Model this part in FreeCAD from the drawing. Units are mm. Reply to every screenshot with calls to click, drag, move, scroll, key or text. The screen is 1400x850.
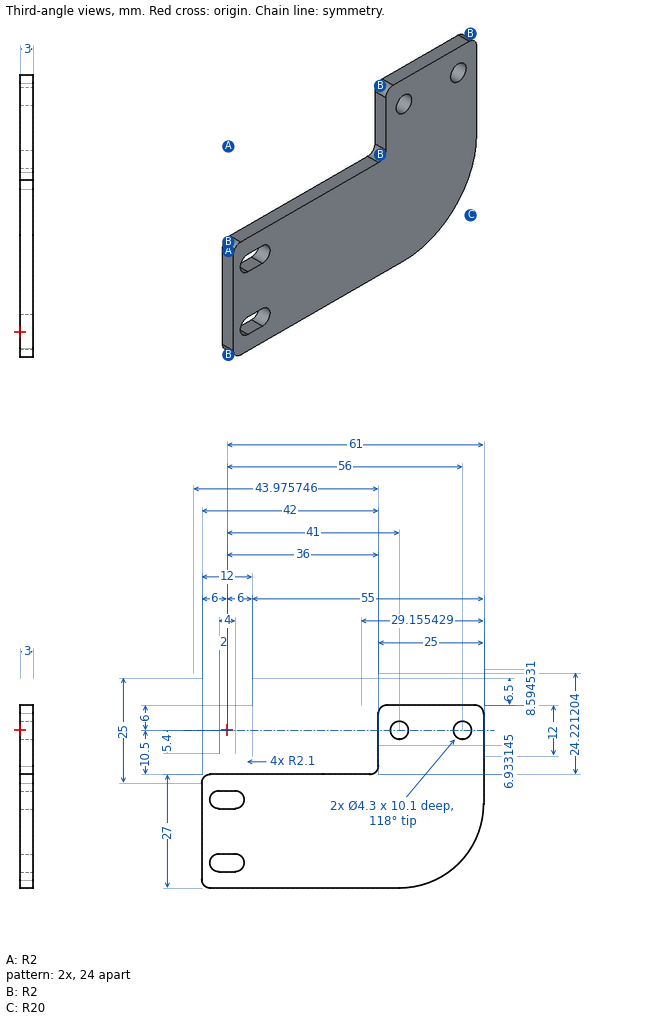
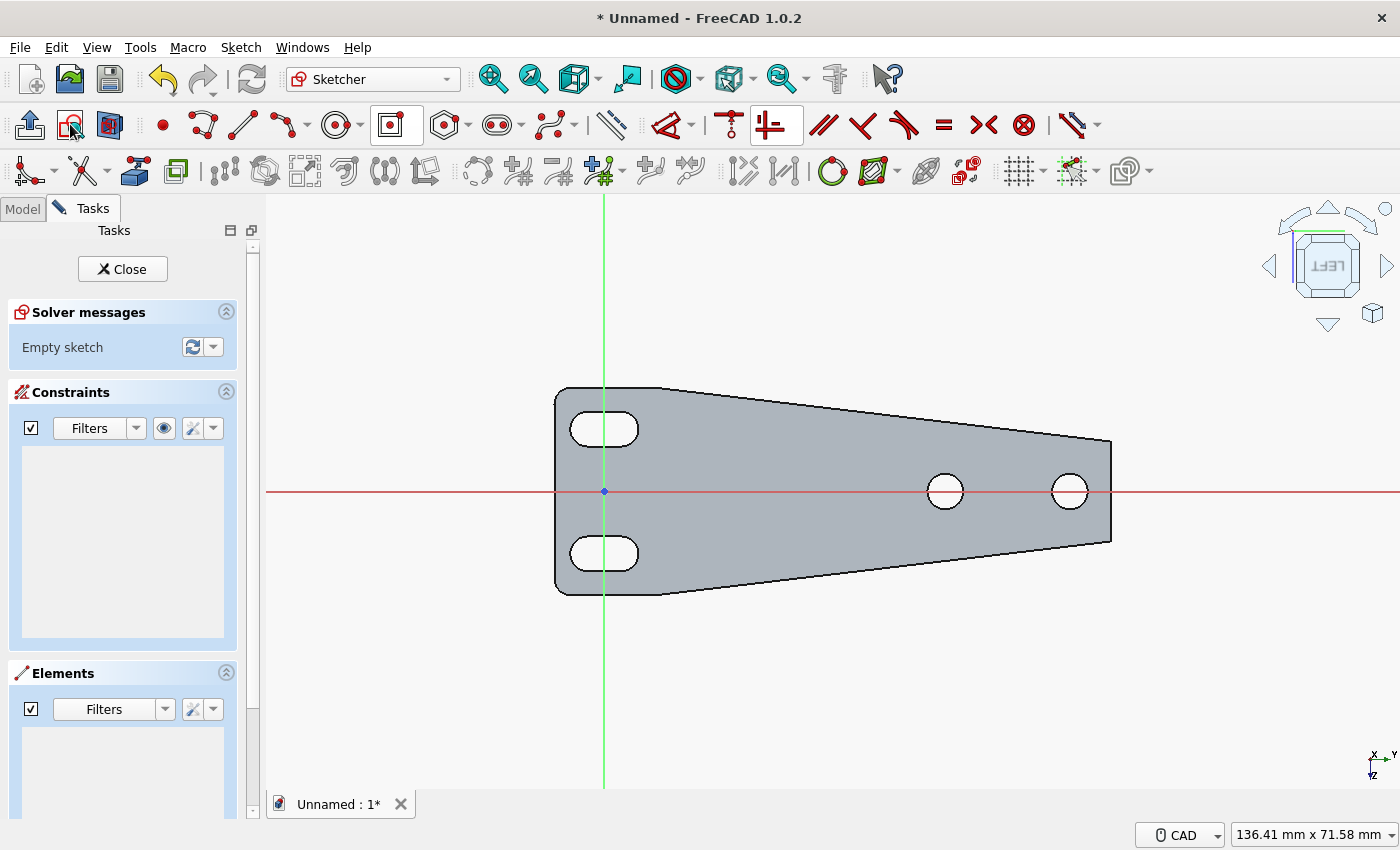
scroll(455, 761, down, 1)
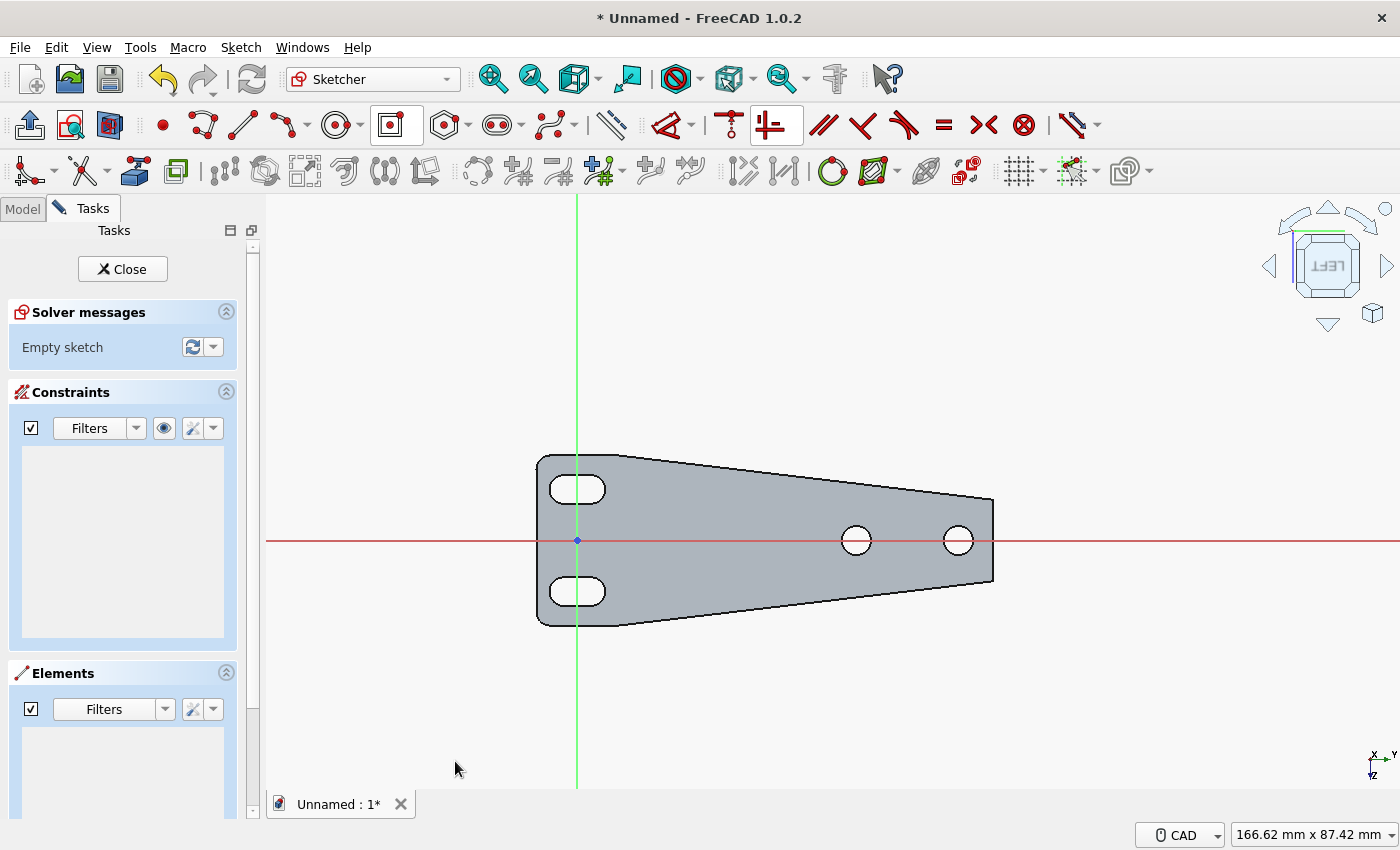
scroll(765, 253, up, 2)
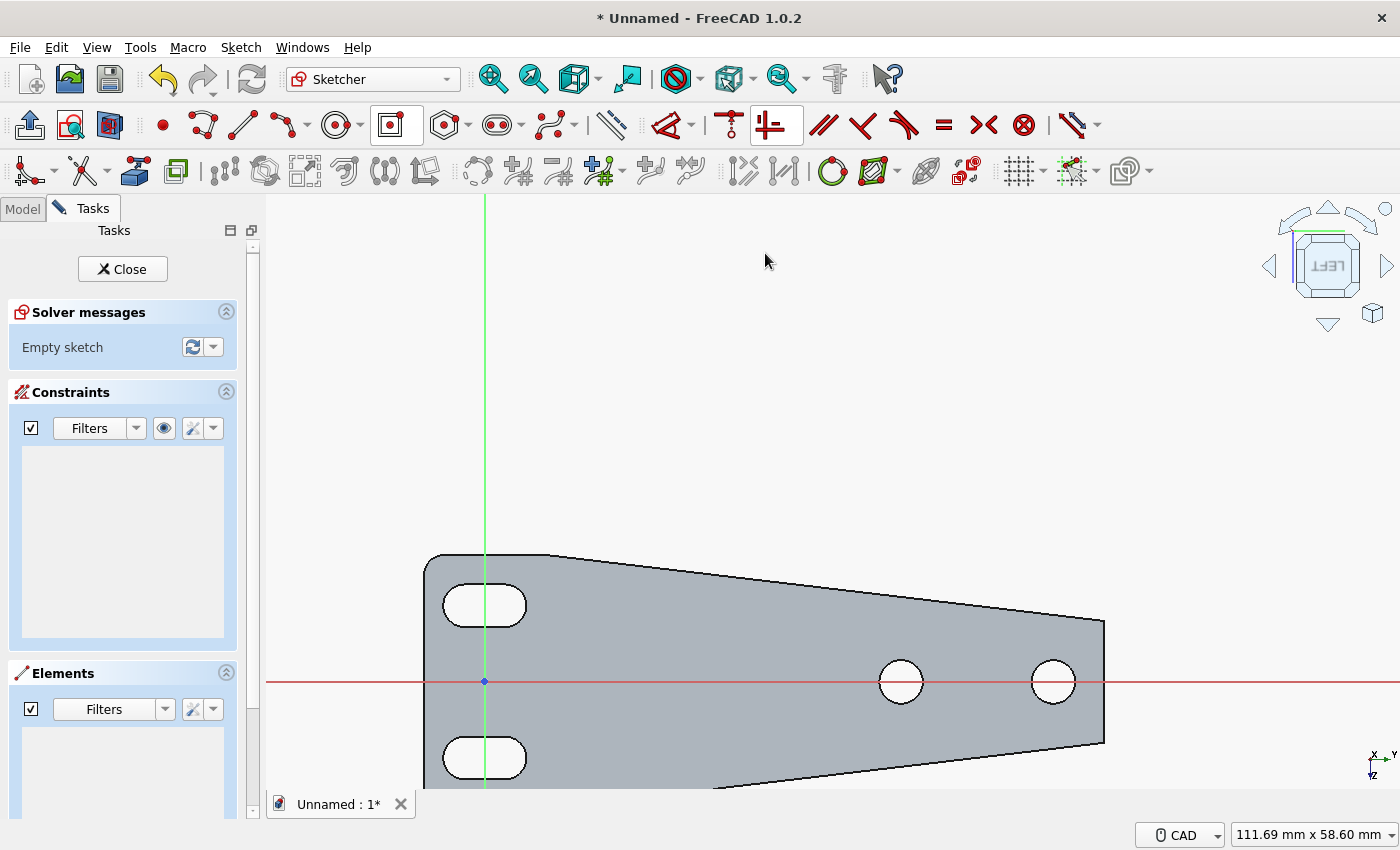
click(204, 126)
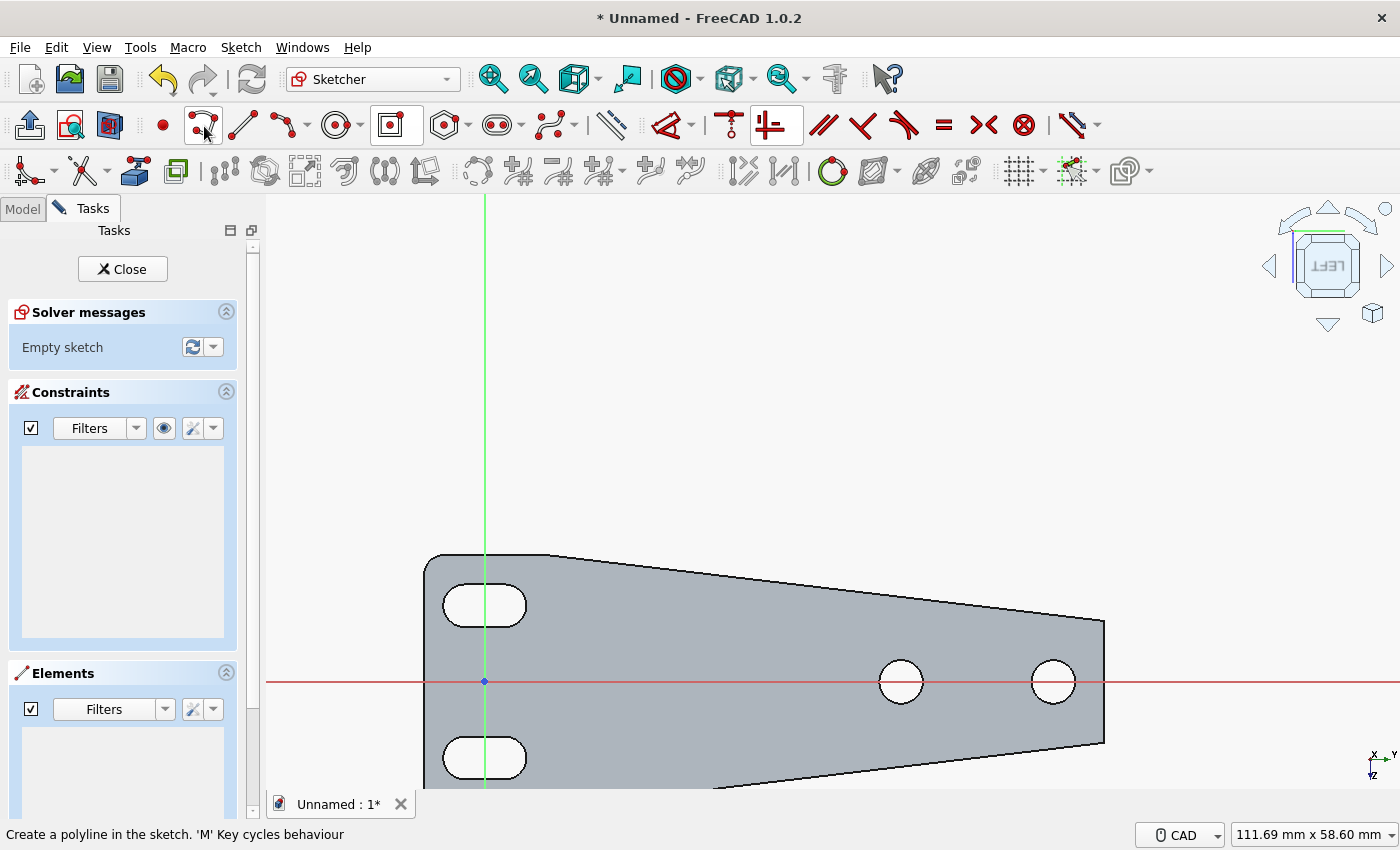
click(424, 575)
click(850, 575)
click(850, 646)
click(1104, 646)
click(1104, 301)
click(424, 301)
click(424, 576)
key(Escape)
key(Escape)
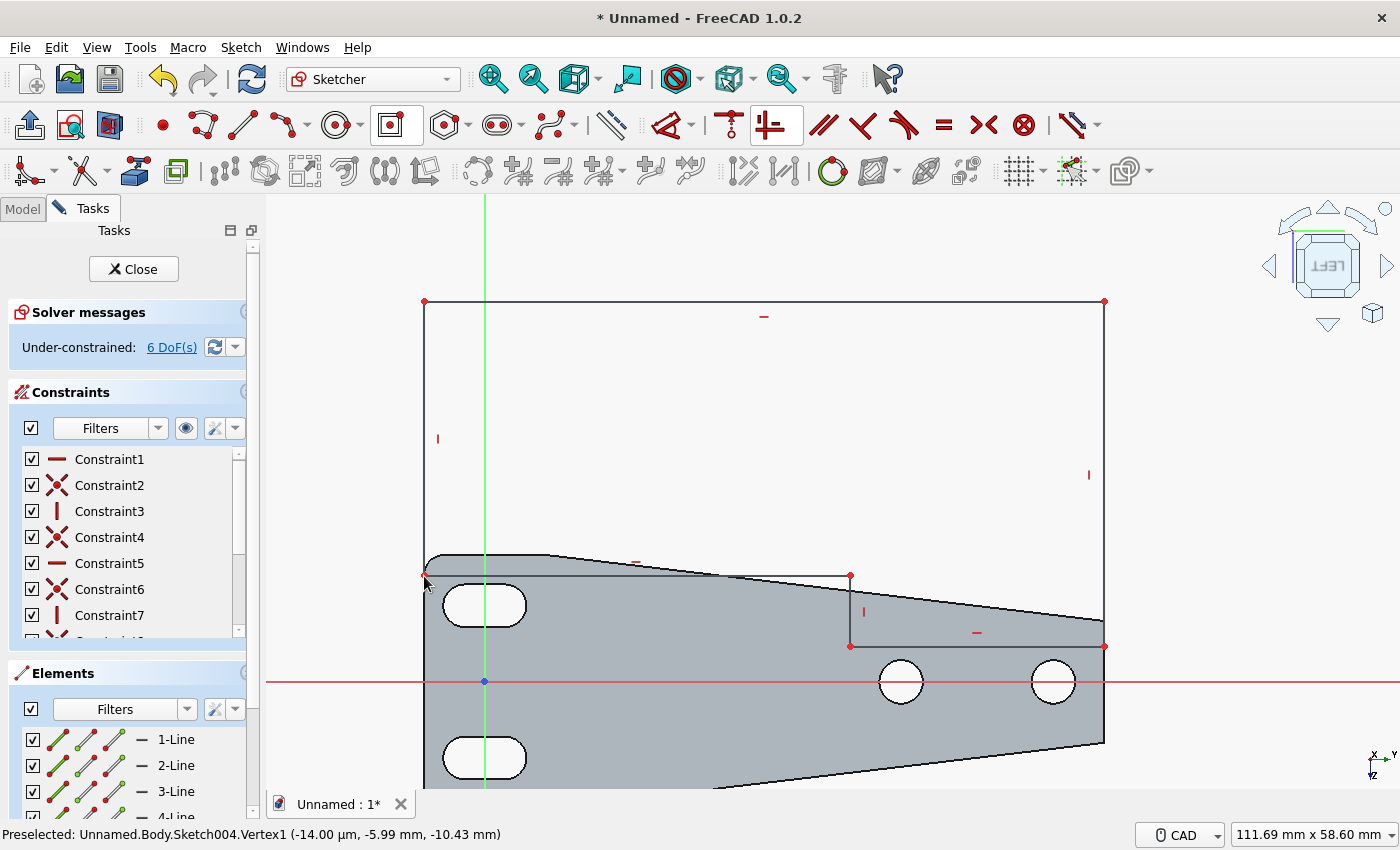
click(666, 126)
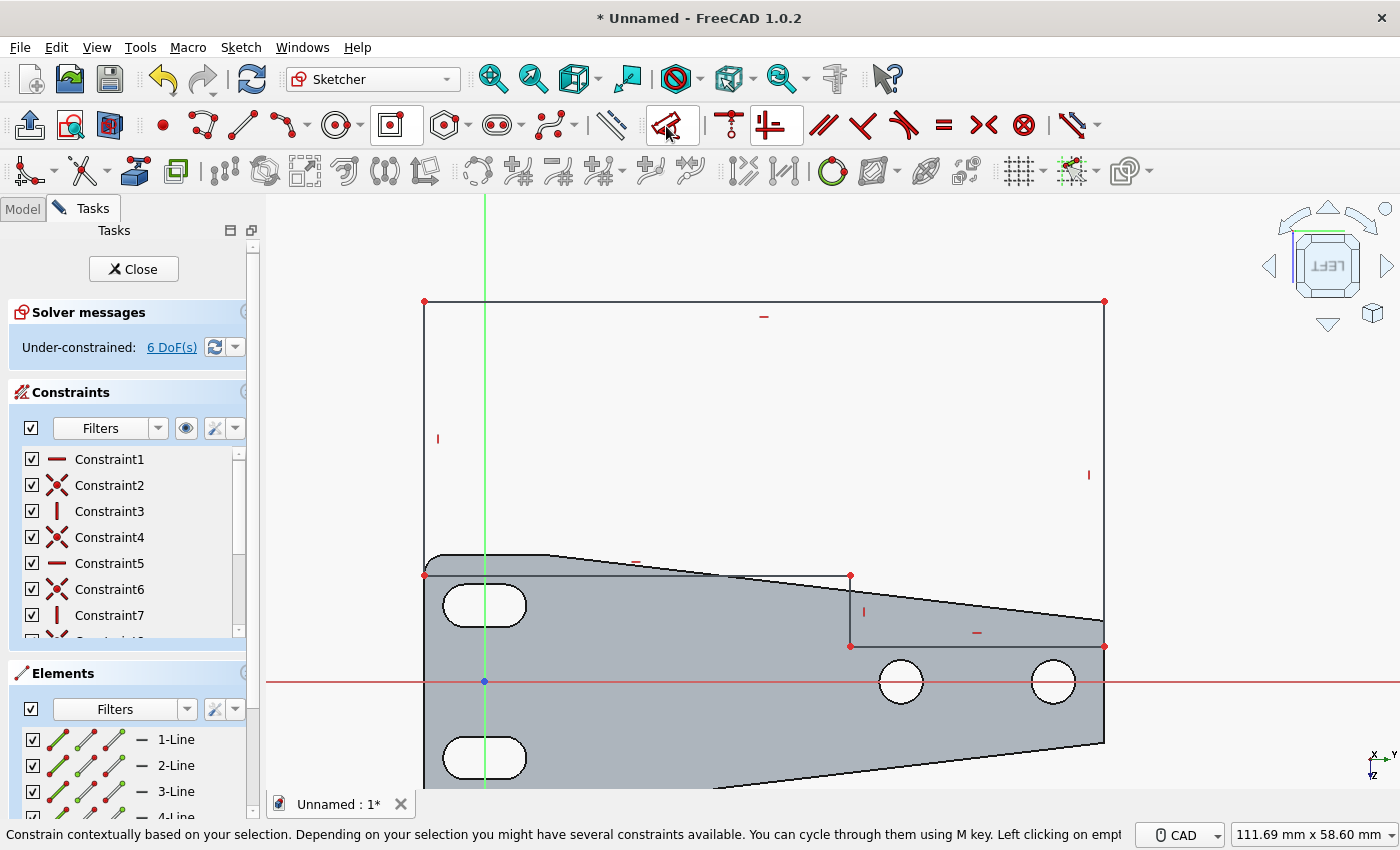
click(552, 576)
click(637, 610)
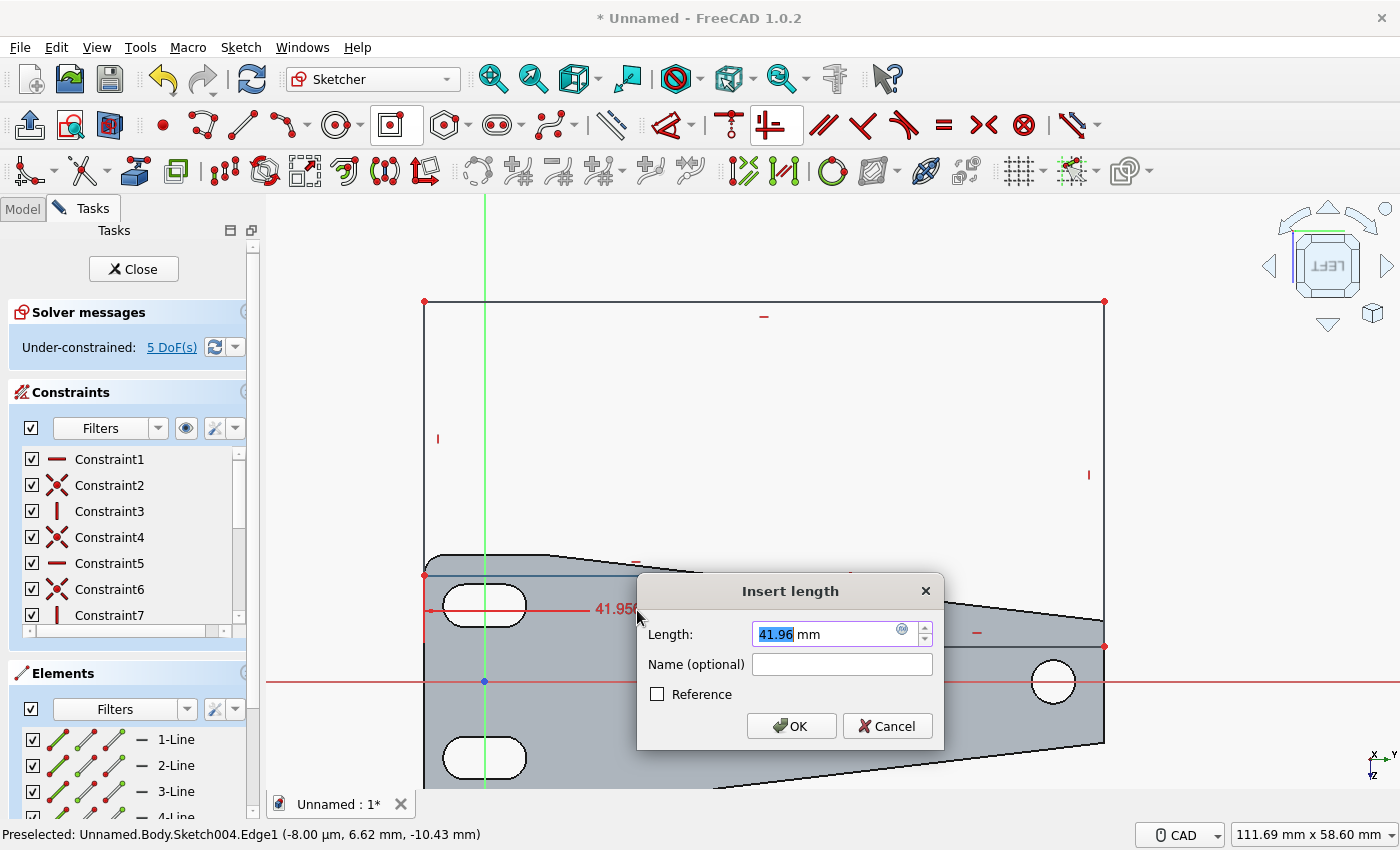
text(42)
key(Return)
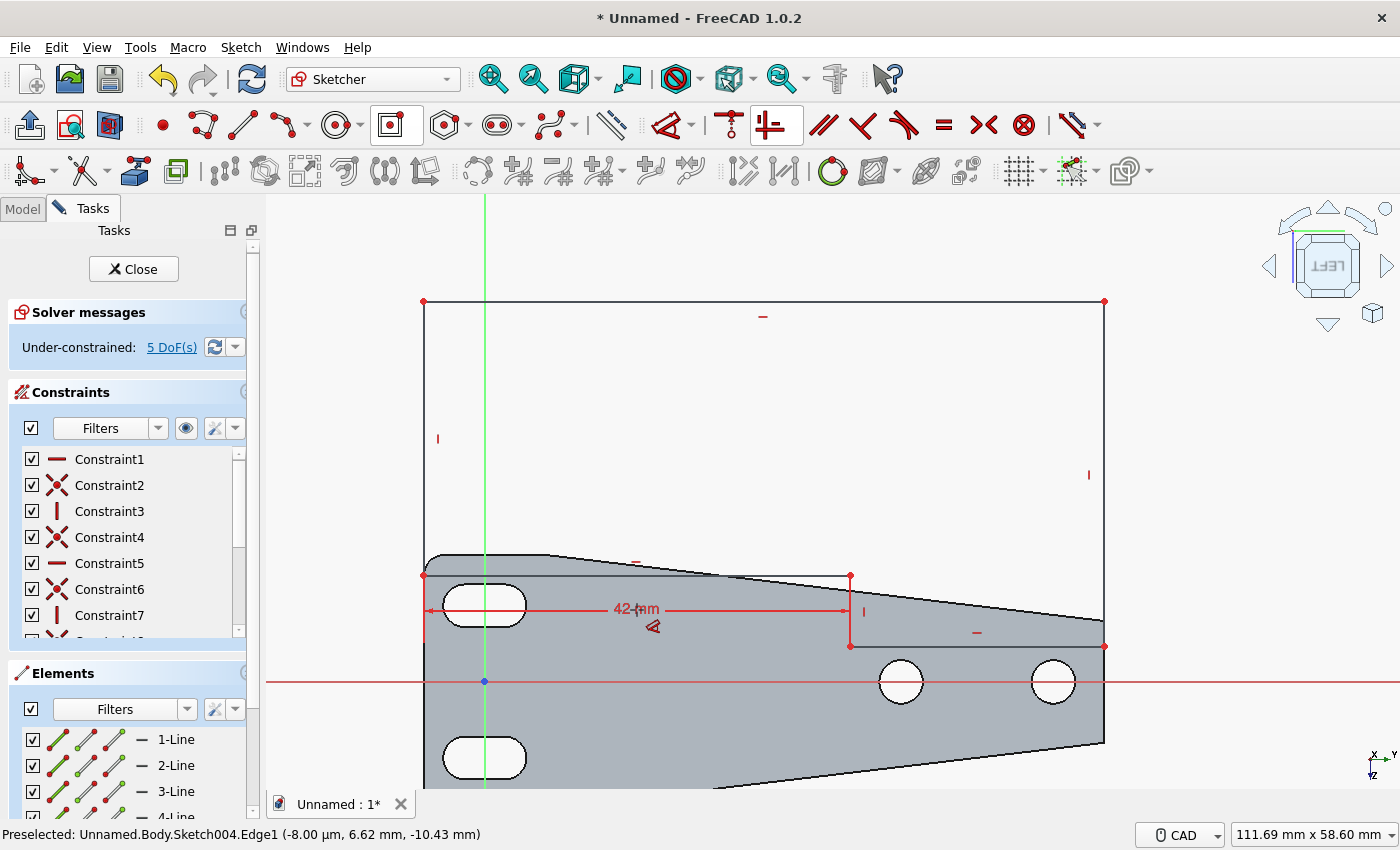
click(926, 647)
click(977, 613)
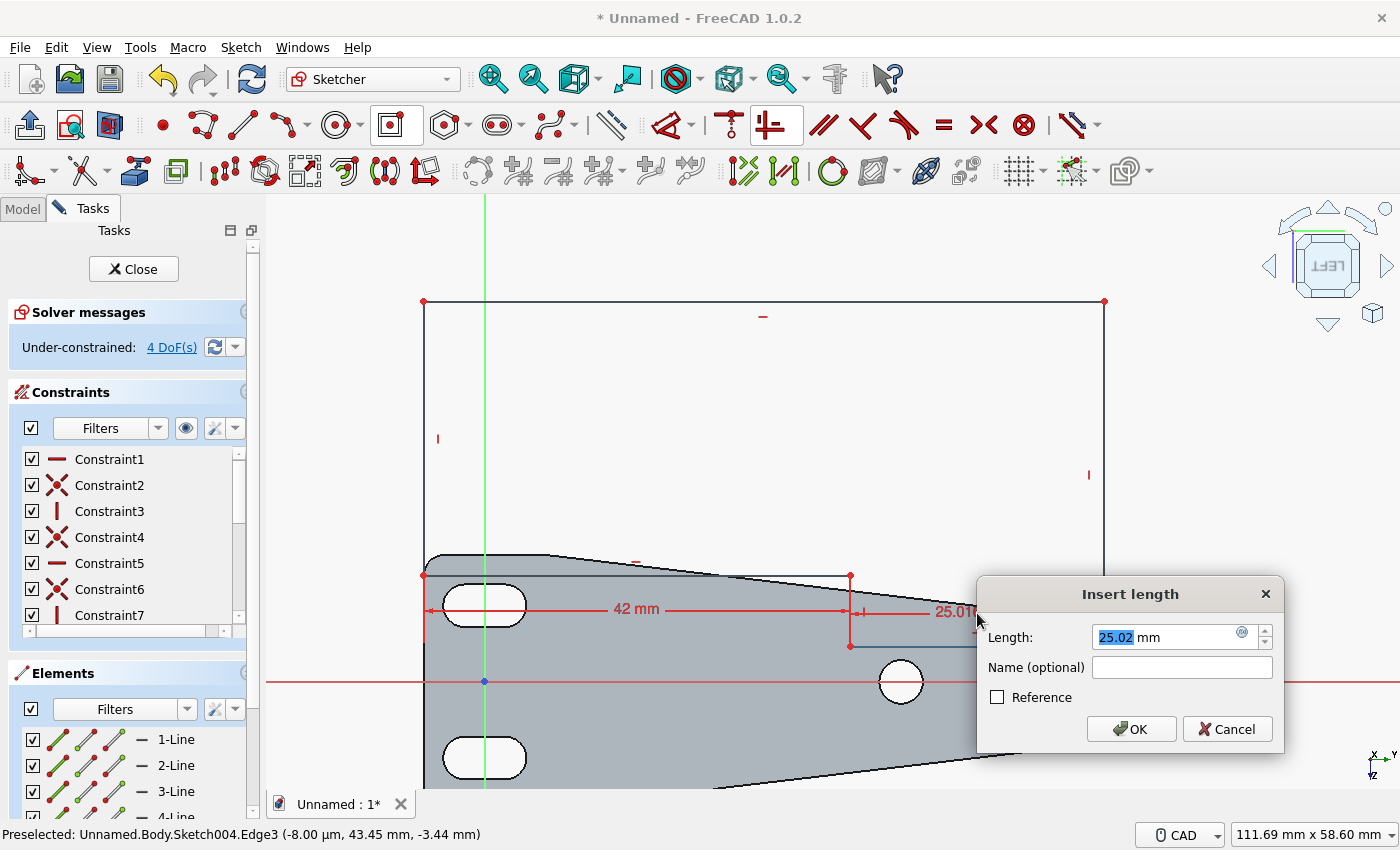
text(25)
key(Return)